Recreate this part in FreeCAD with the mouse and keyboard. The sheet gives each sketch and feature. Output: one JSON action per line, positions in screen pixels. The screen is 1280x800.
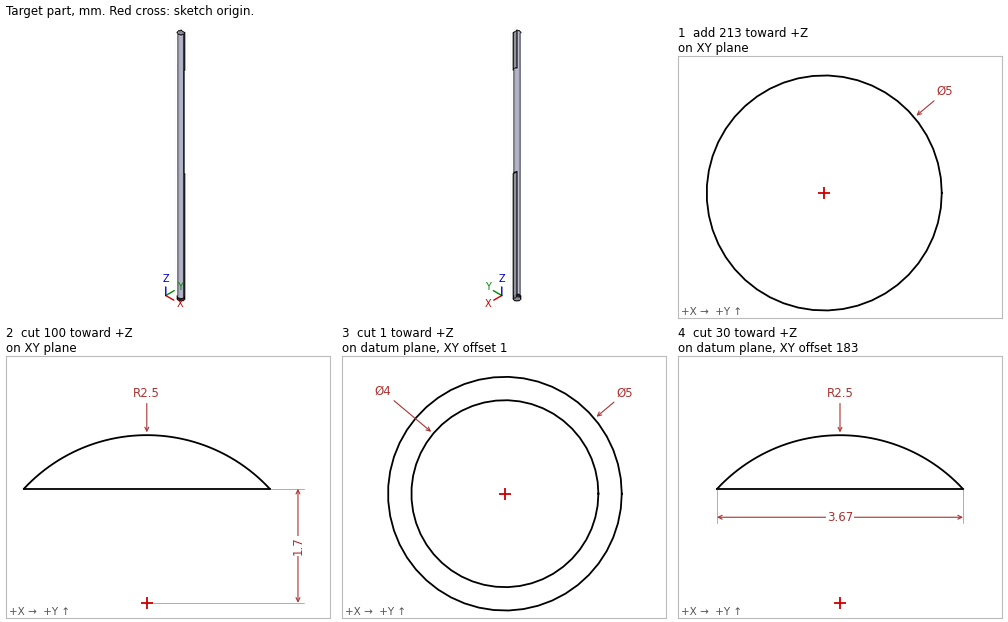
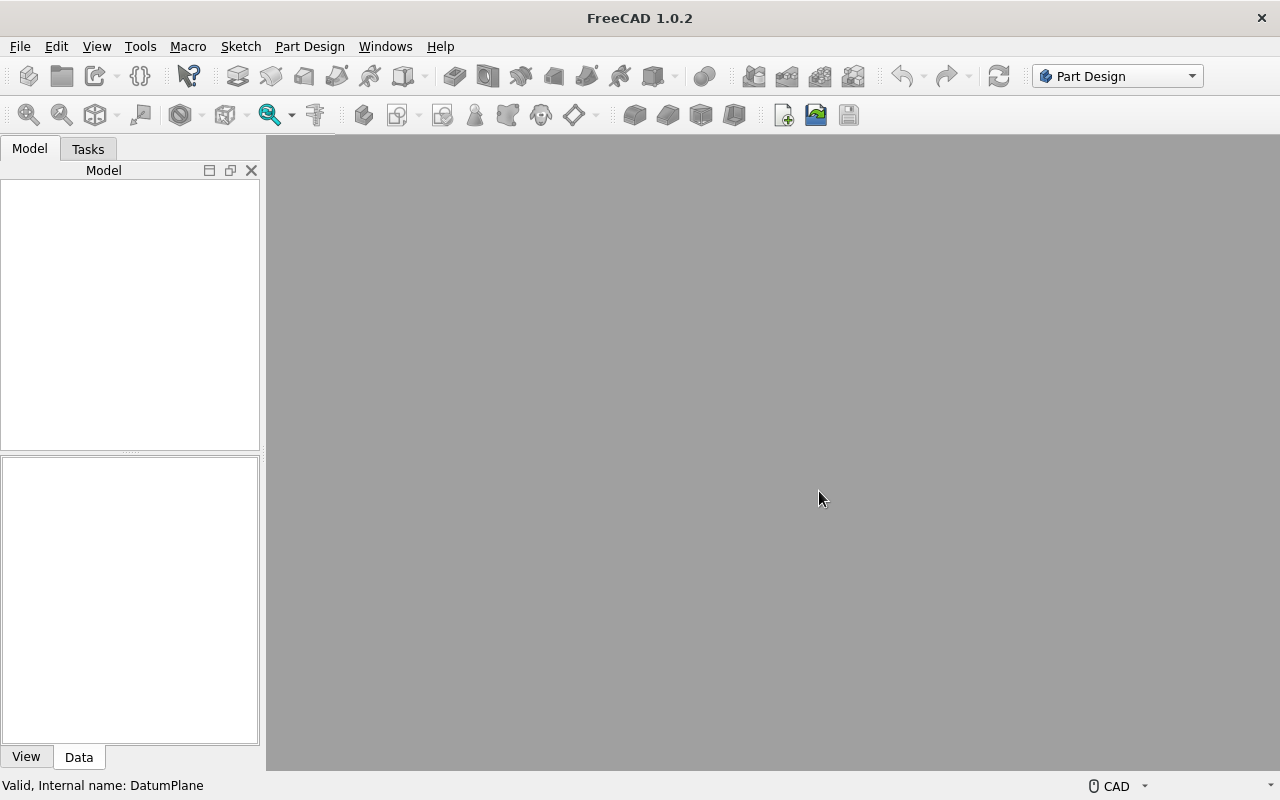
{"action": "key", "text": "ctrl+n"}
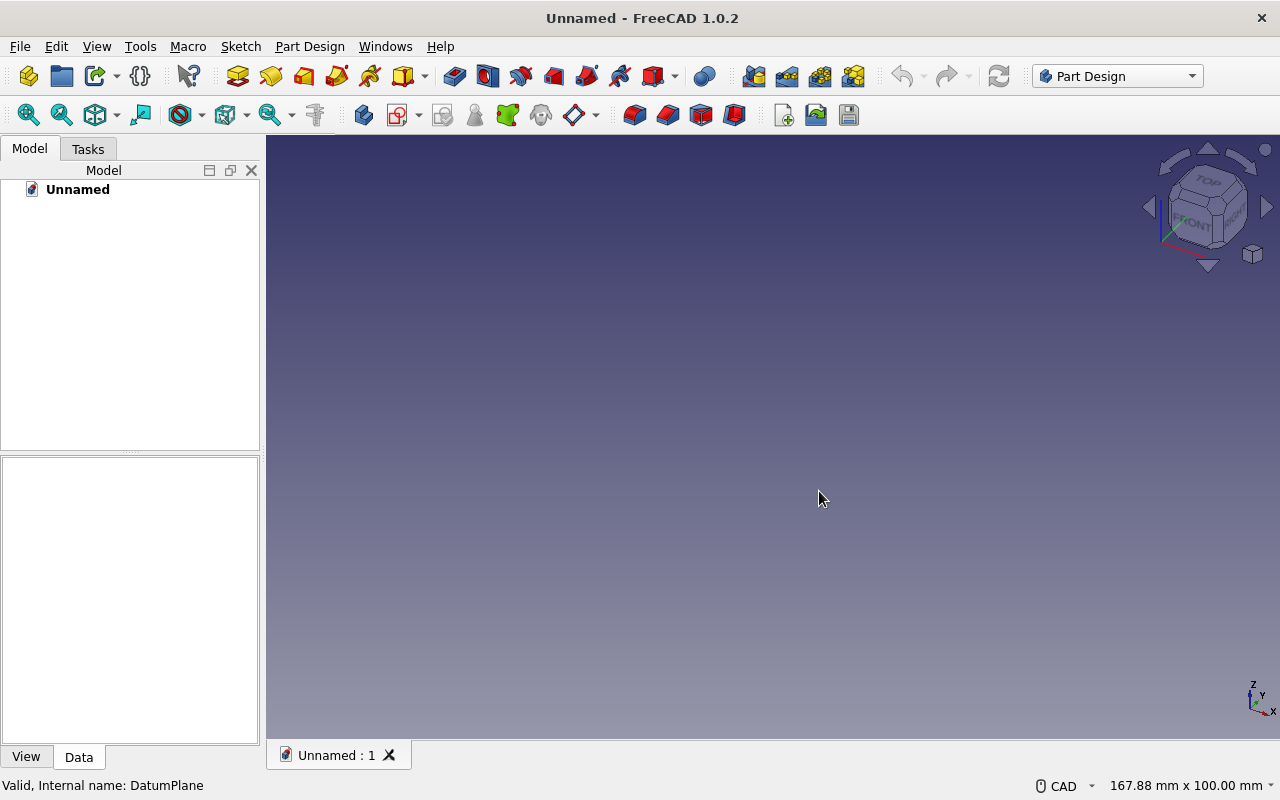
{"action": "left_click", "coordinate": [396, 116]}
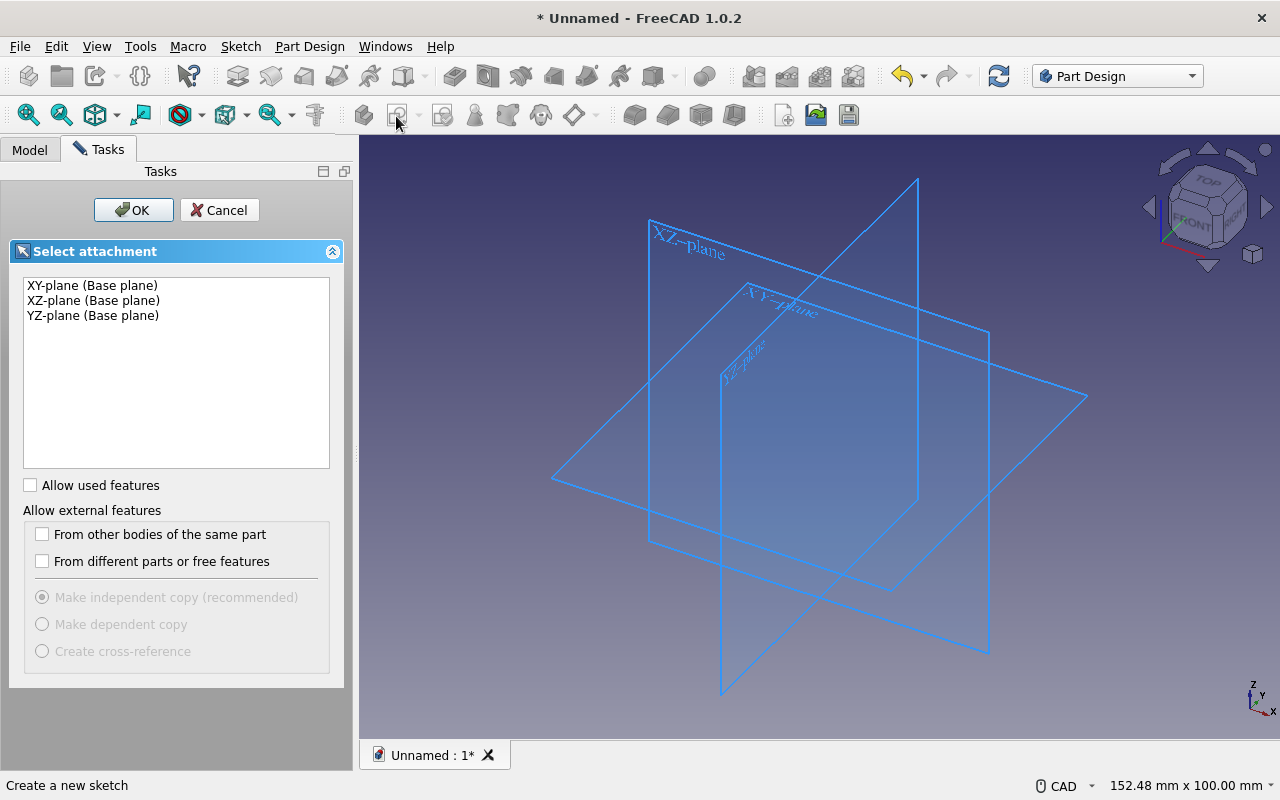
{"action": "left_click", "coordinate": [84, 286]}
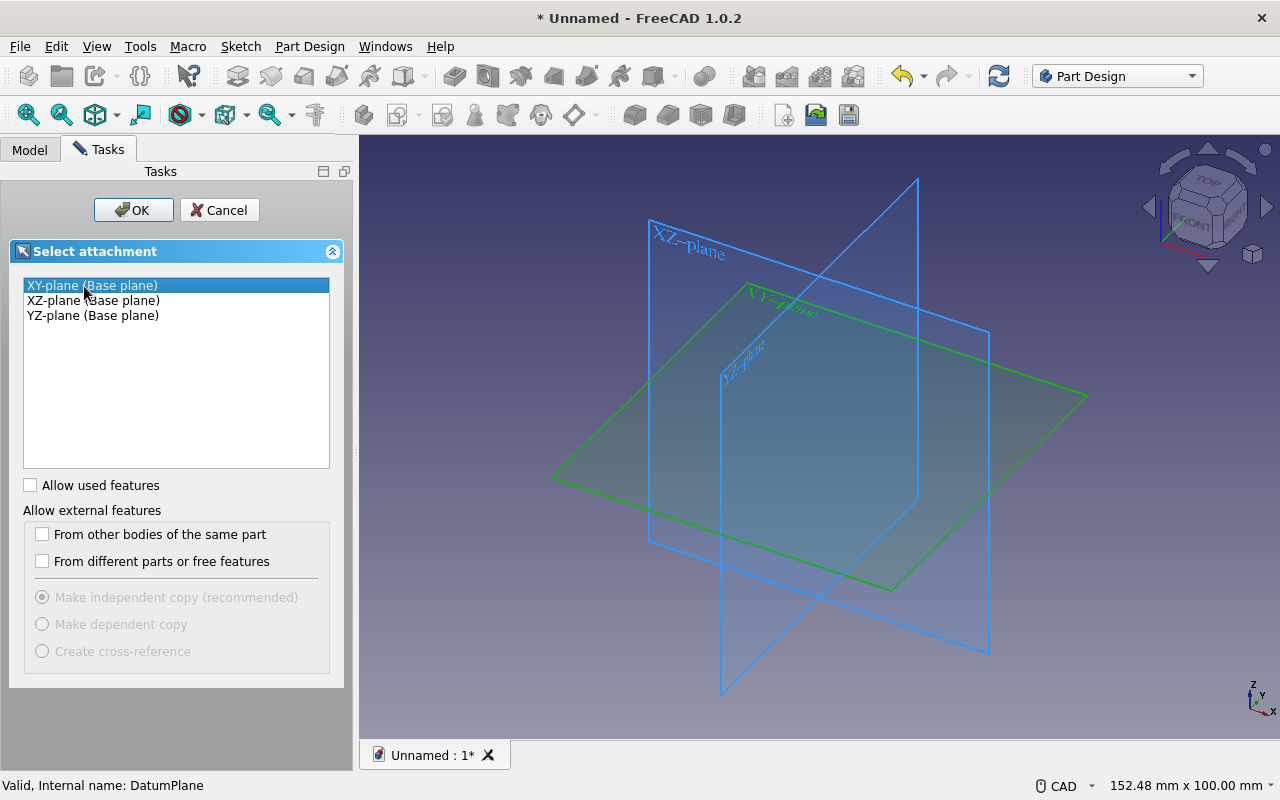
{"action": "left_click", "coordinate": [134, 210]}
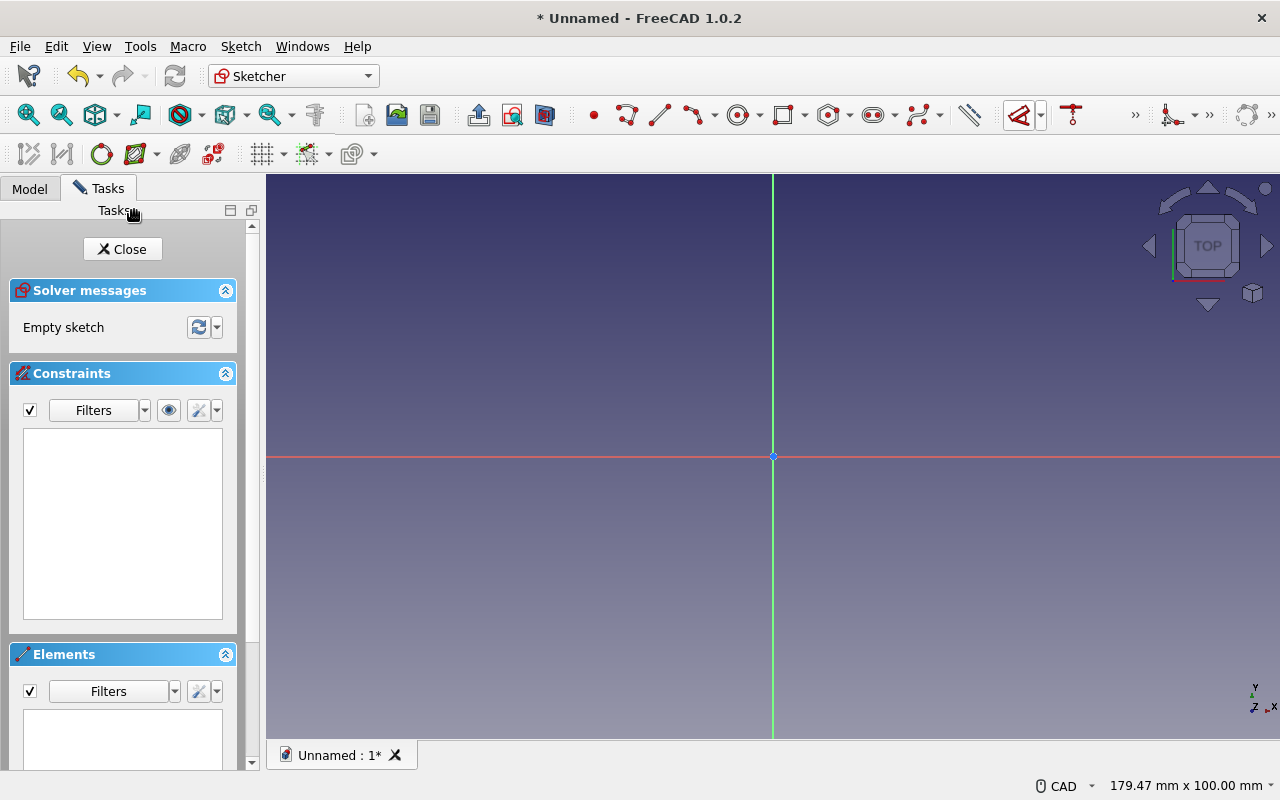
{"action": "scroll", "coordinate": [778, 456], "scroll_direction": "up", "scroll_amount": 13}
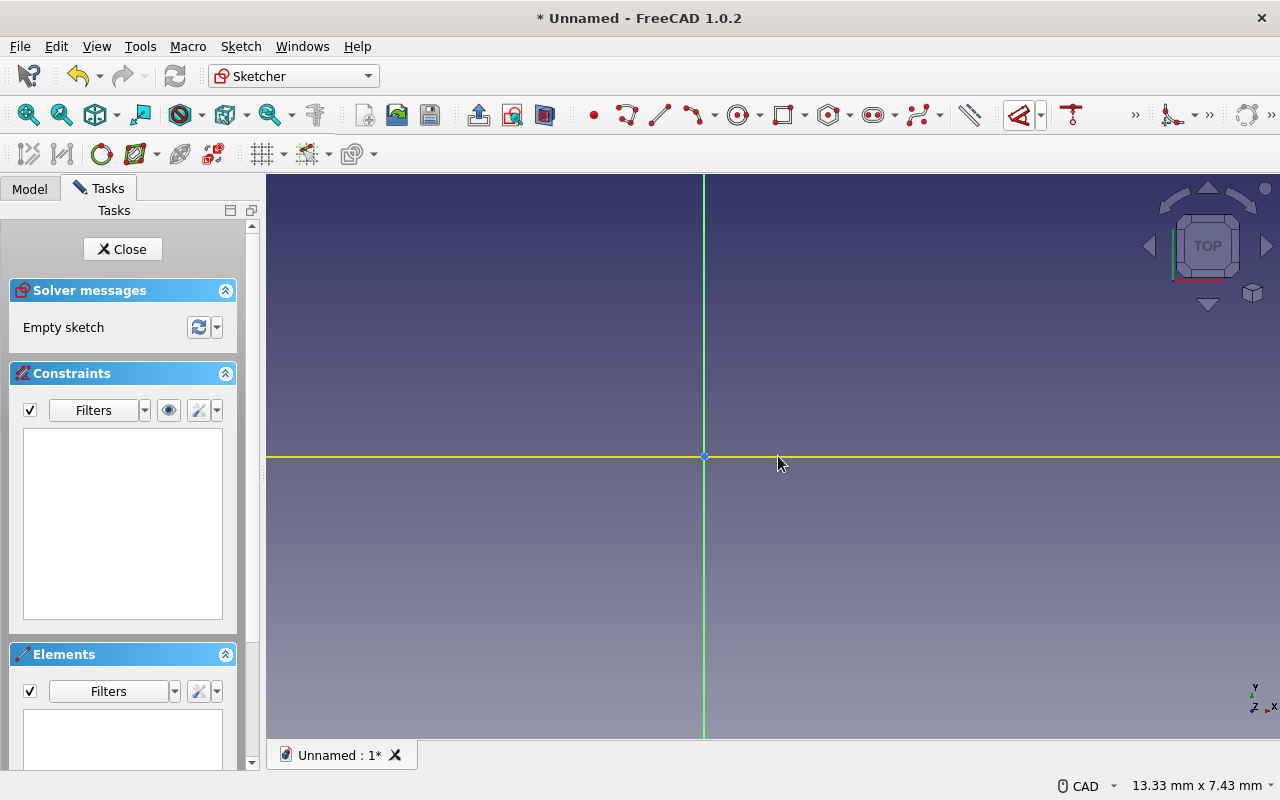
{"action": "key", "text": "g c"}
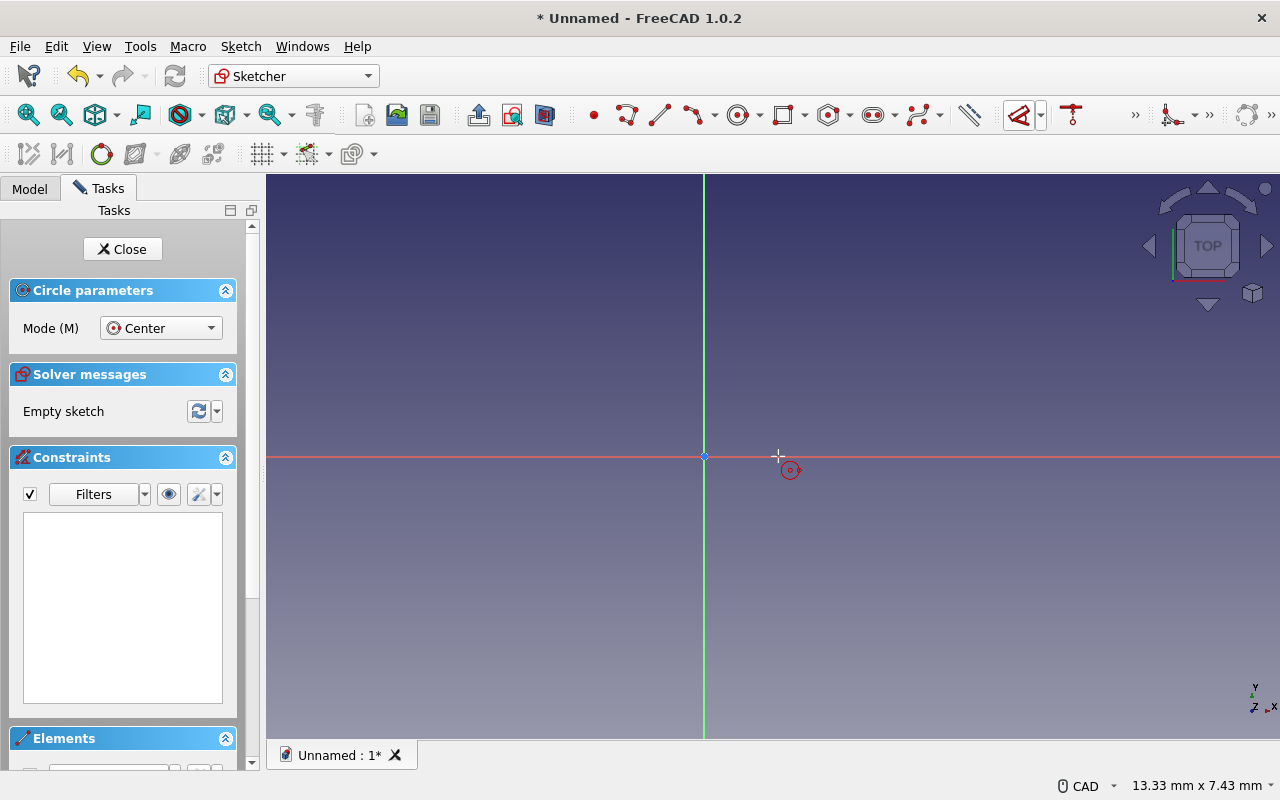
{"action": "left_click", "coordinate": [704, 456]}
{"action": "mouse_move", "coordinate": [839, 322]}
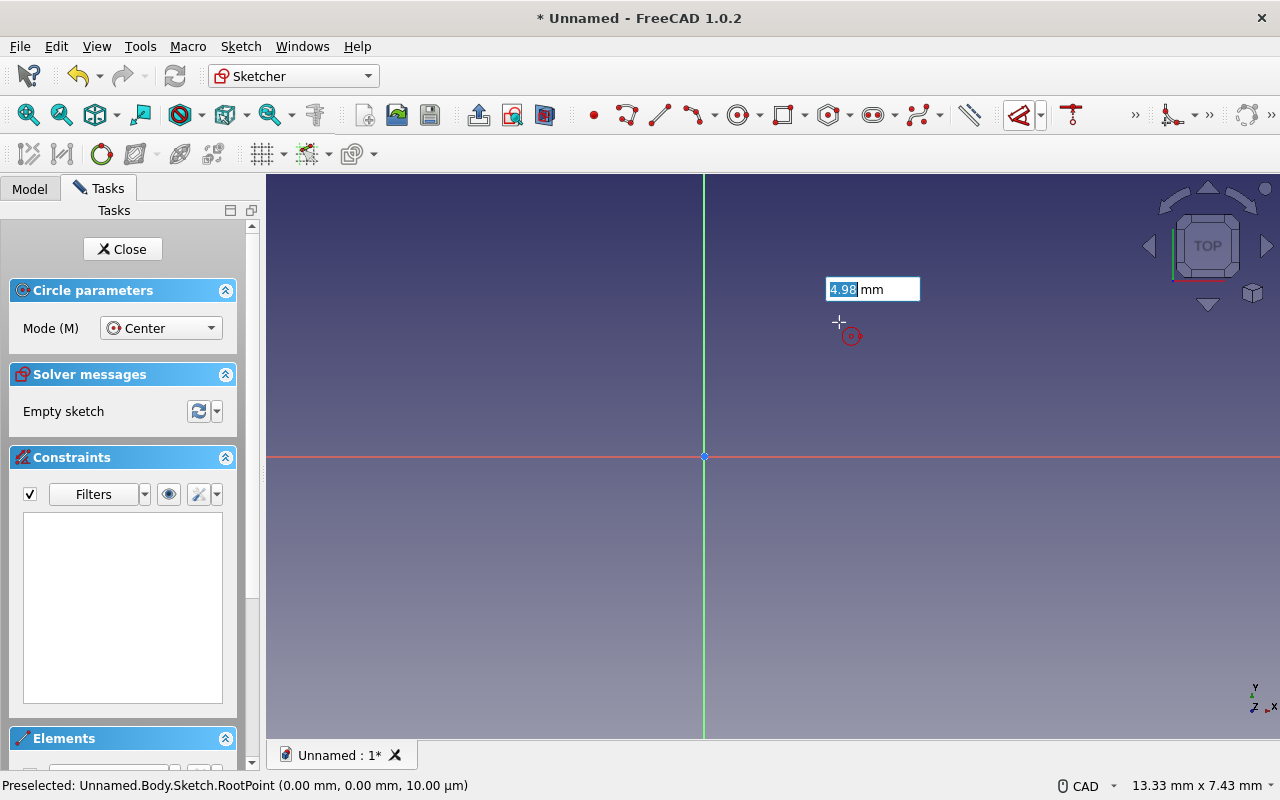
{"action": "type", "text": "5"}
{"action": "key", "text": "Return"}
{"action": "key", "text": "Escape"}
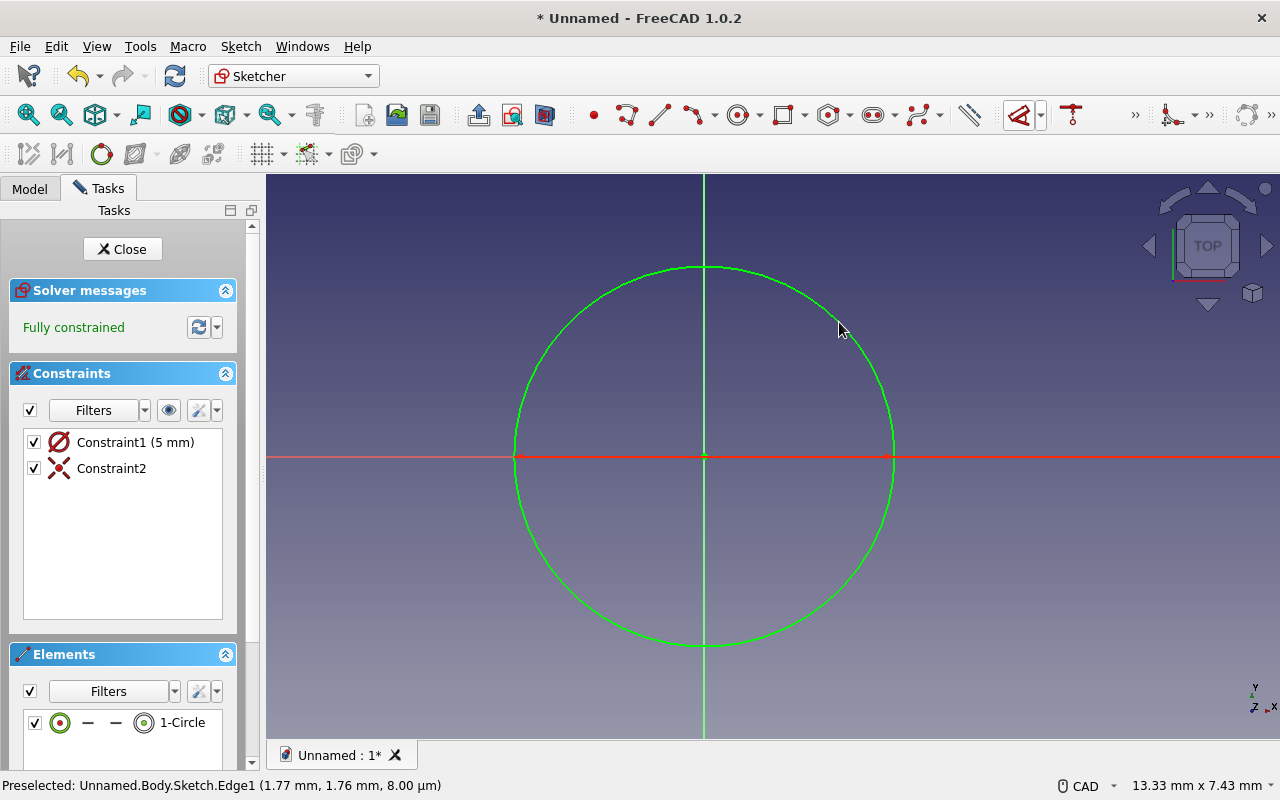
{"action": "left_click", "coordinate": [123, 249]}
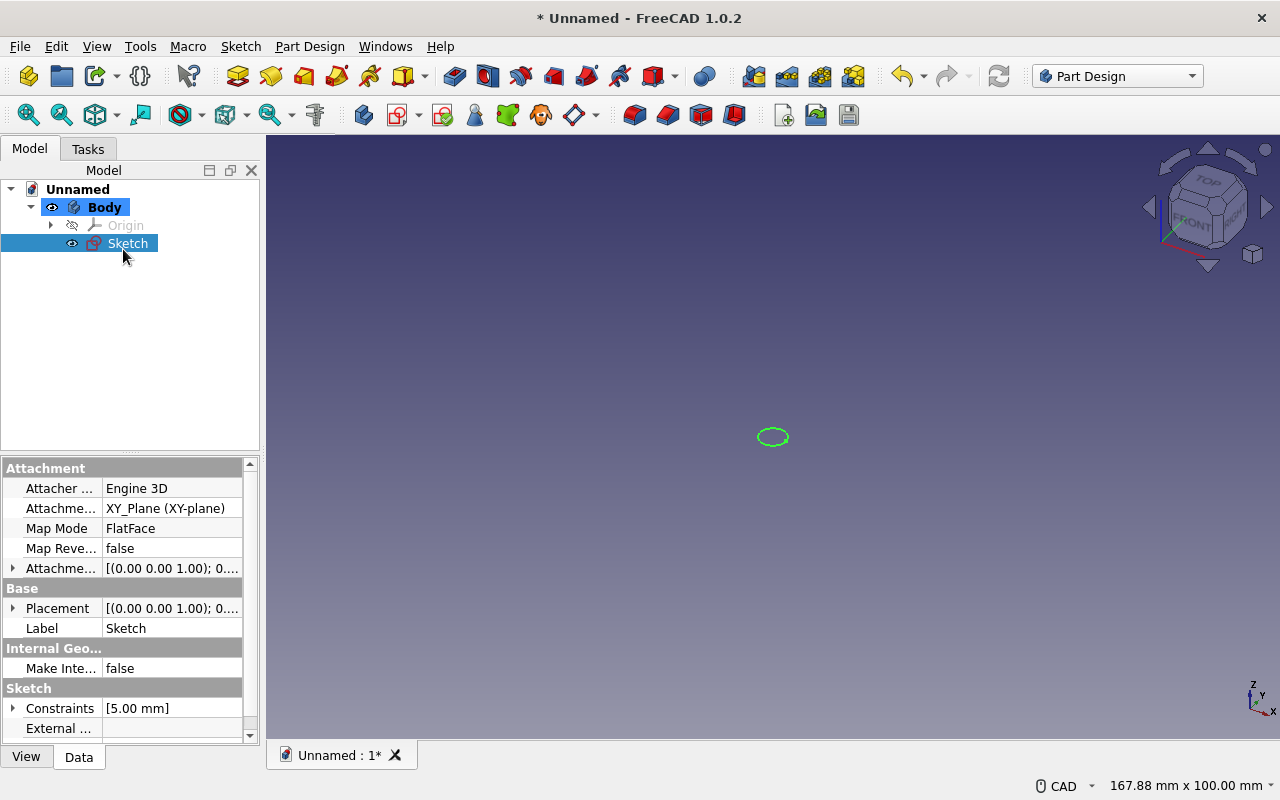
{"action": "left_click", "coordinate": [238, 76]}